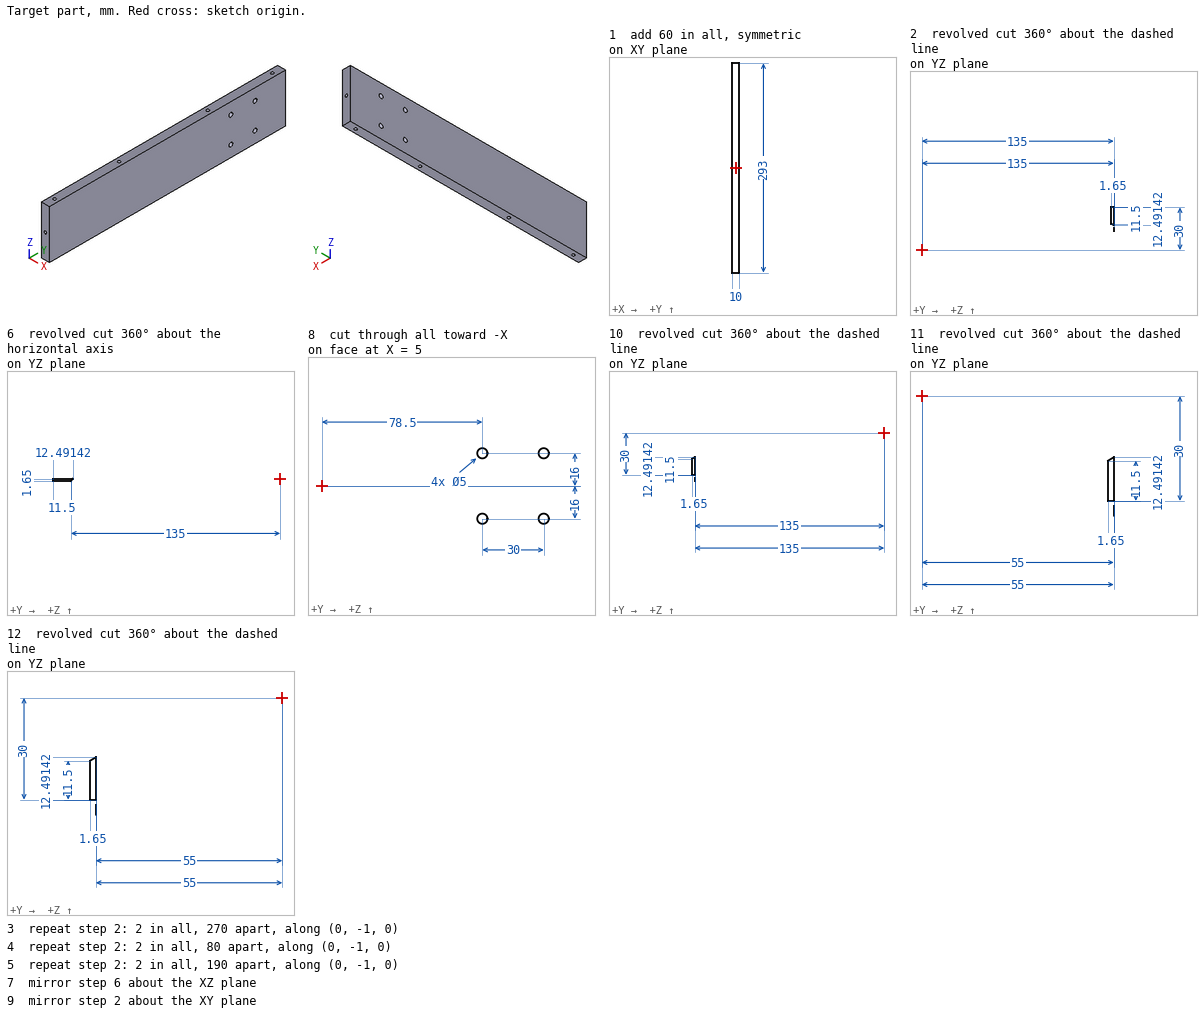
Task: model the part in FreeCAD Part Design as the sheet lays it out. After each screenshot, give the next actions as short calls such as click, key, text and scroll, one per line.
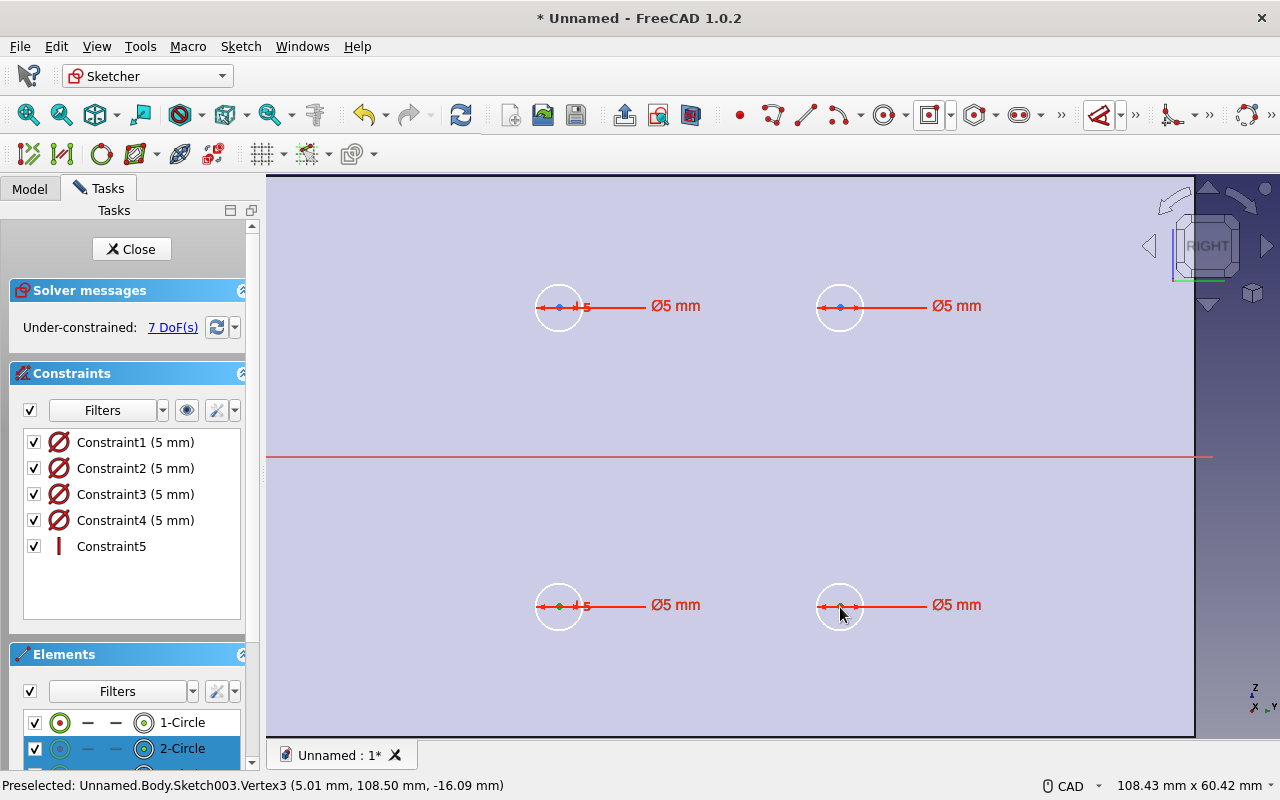
key(h)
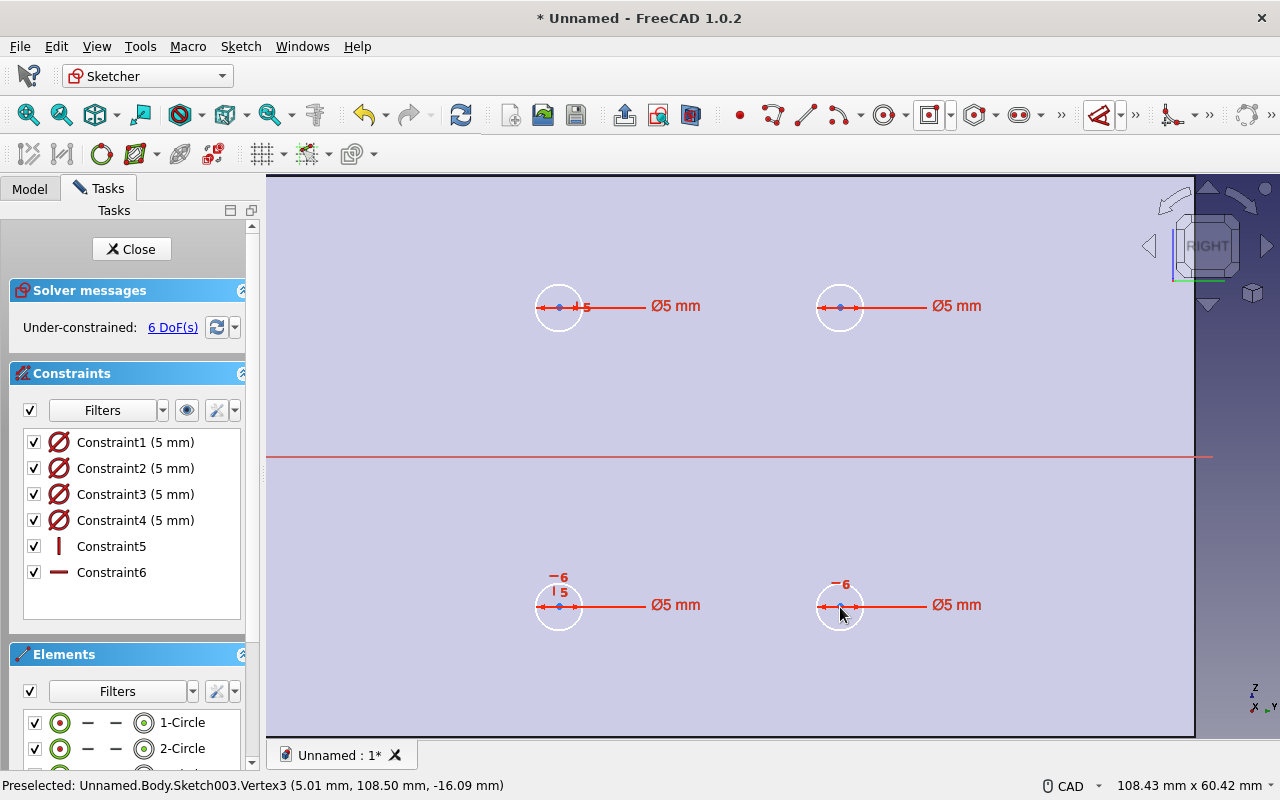
click(840, 607)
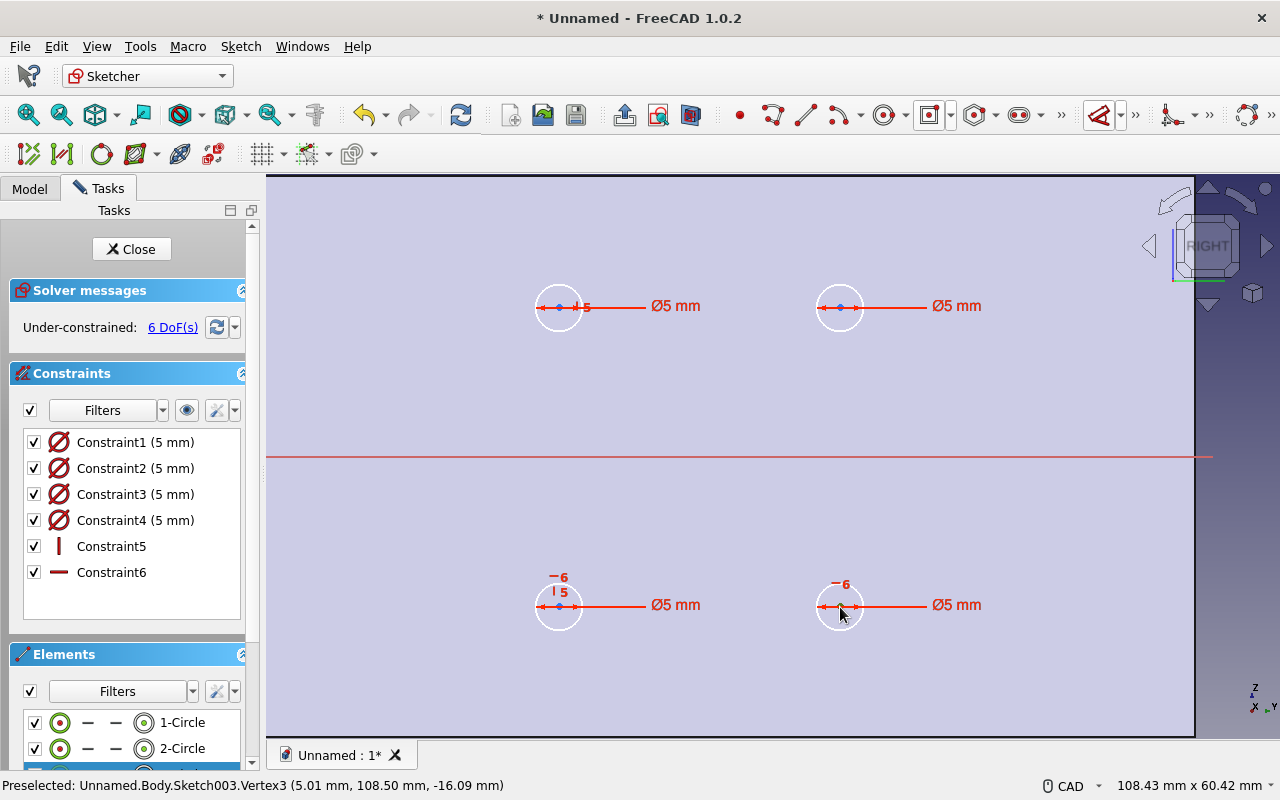
click(840, 308)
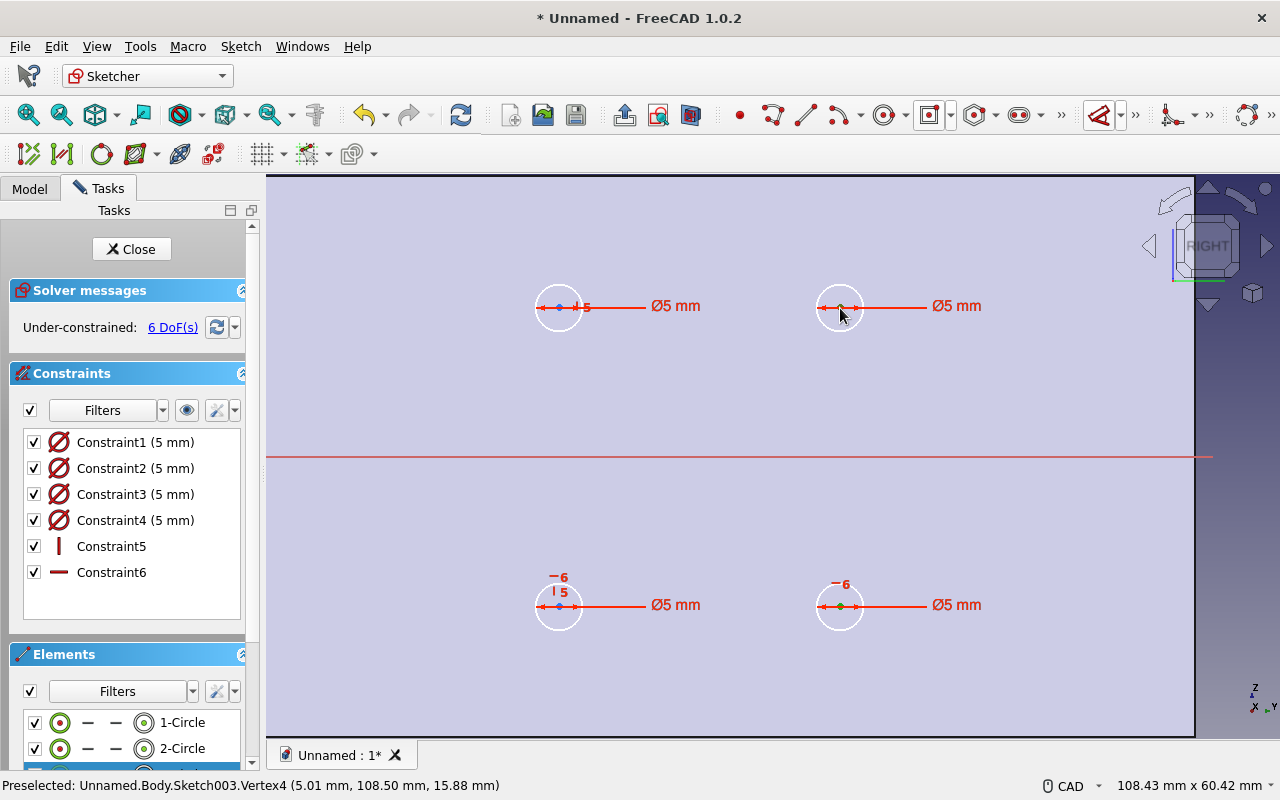
key(v)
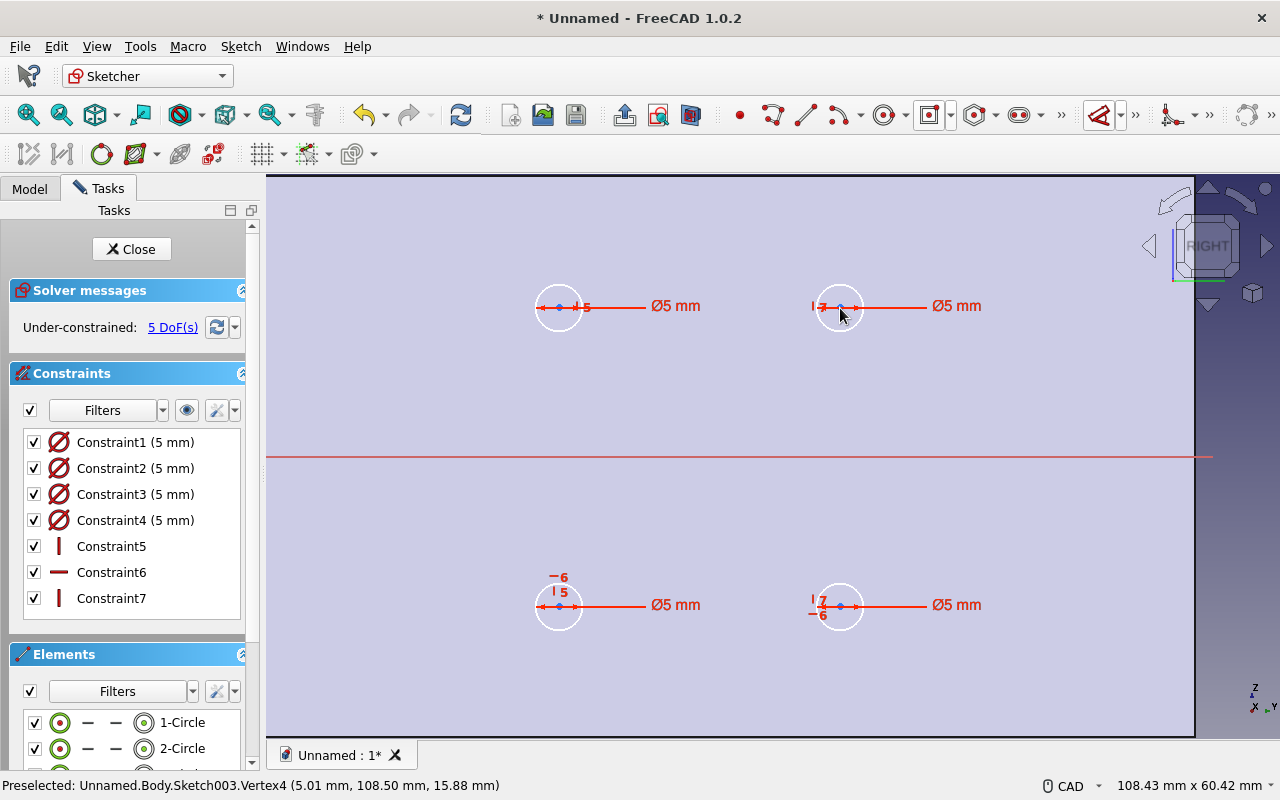
click(559, 308)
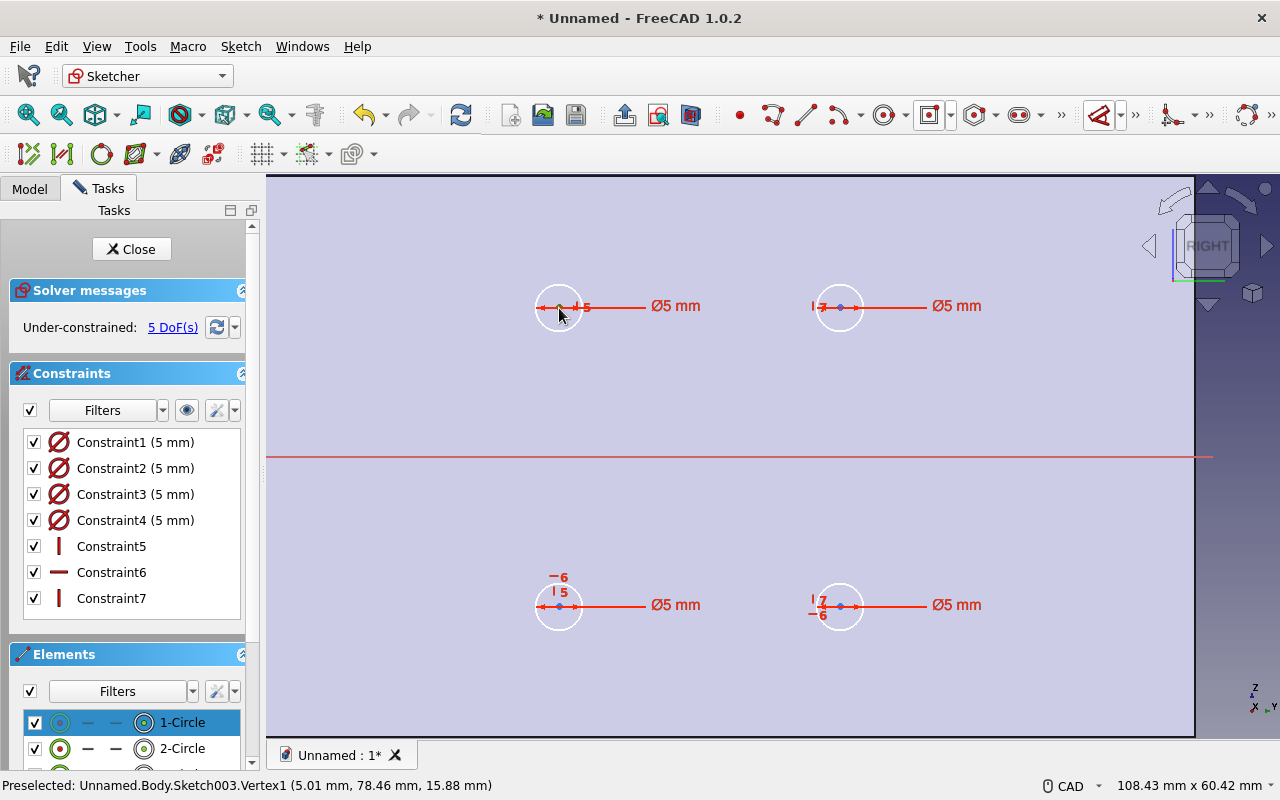
click(840, 308)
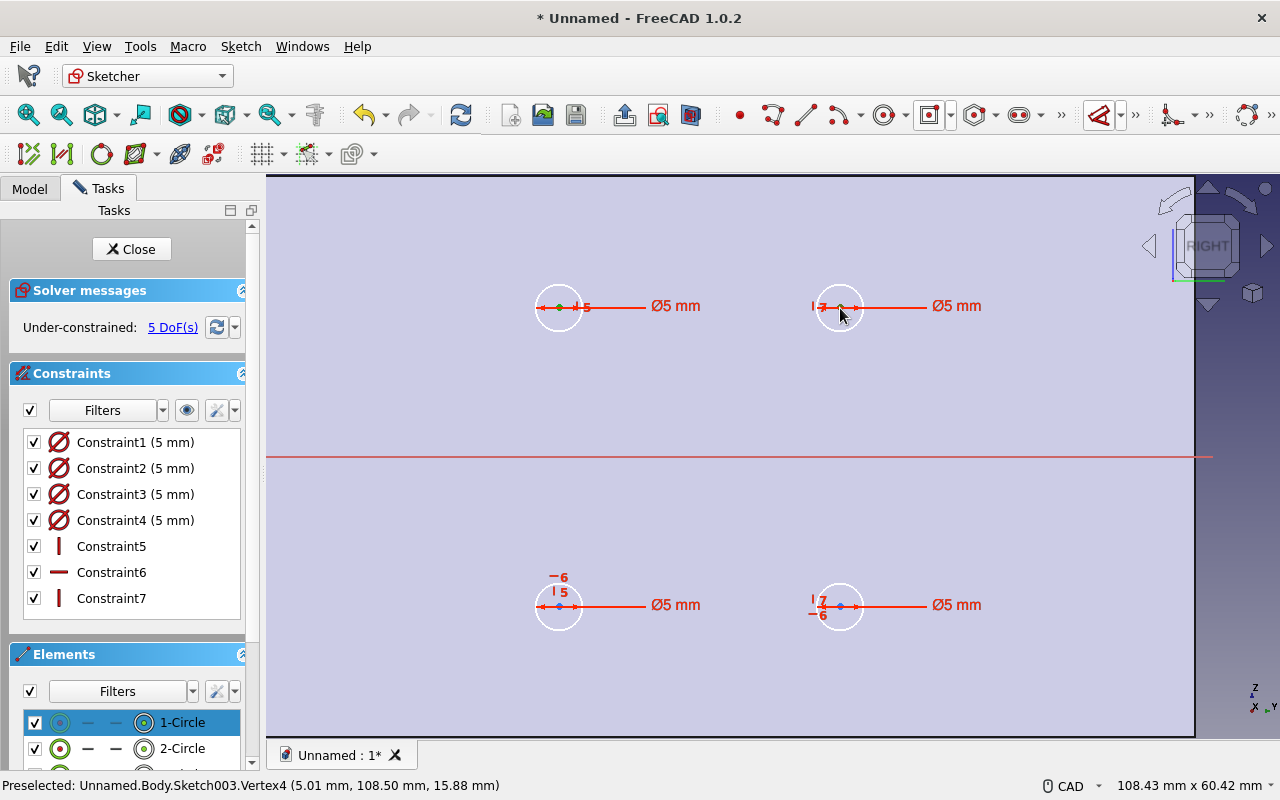
key(h)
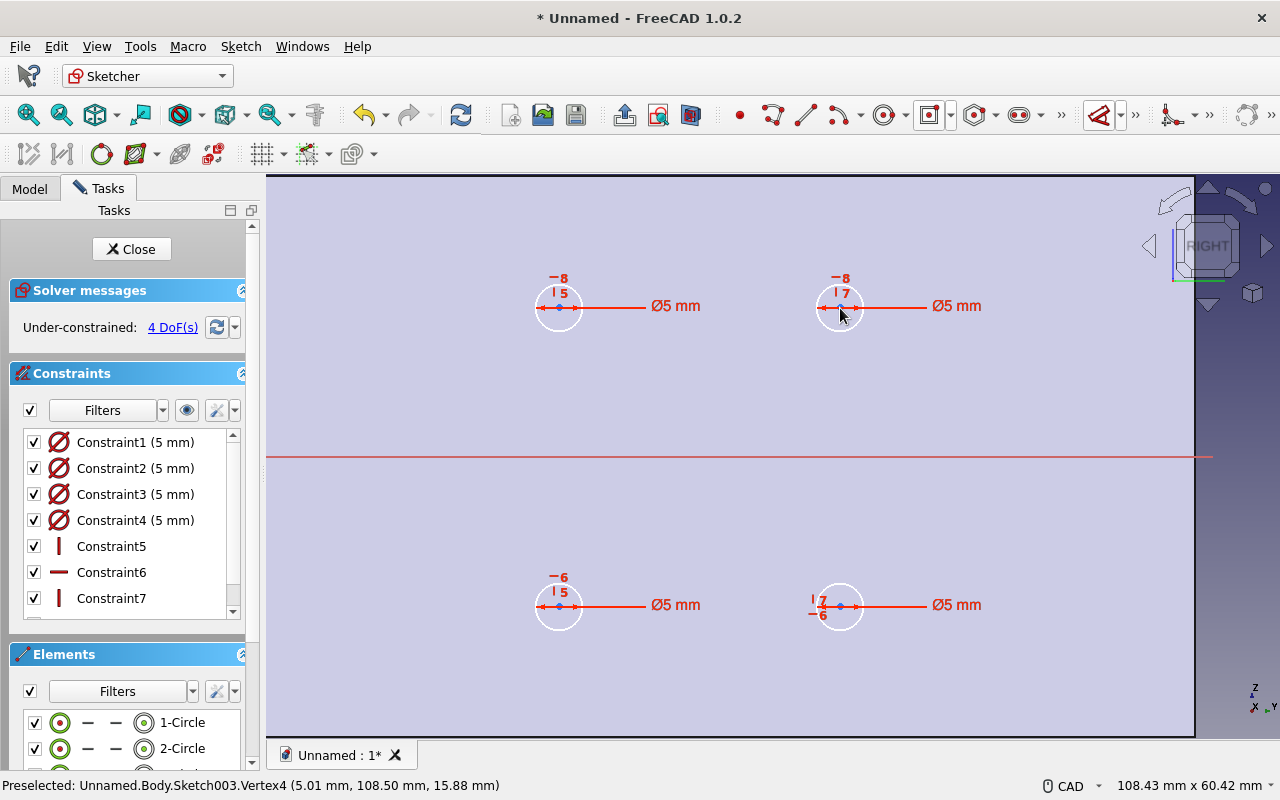
click(559, 308)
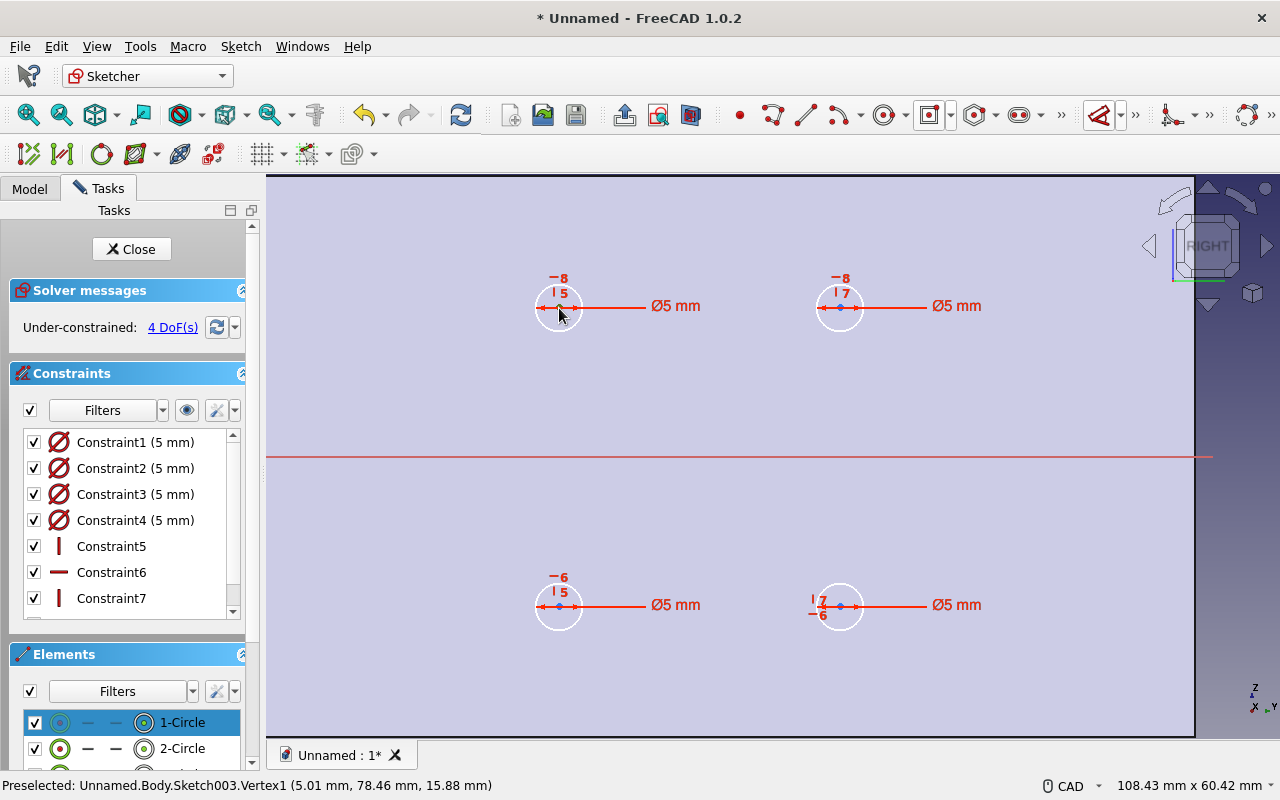
click(1120, 116)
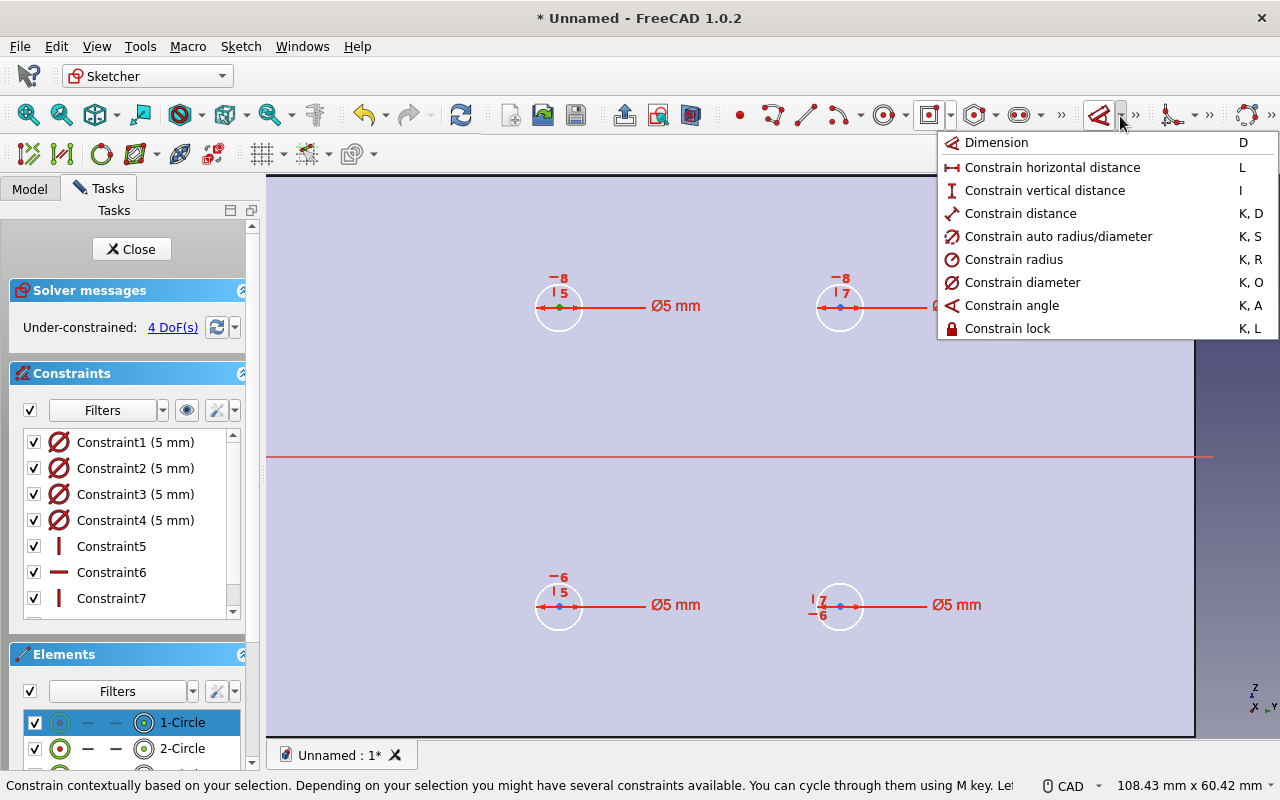
click(1108, 190)